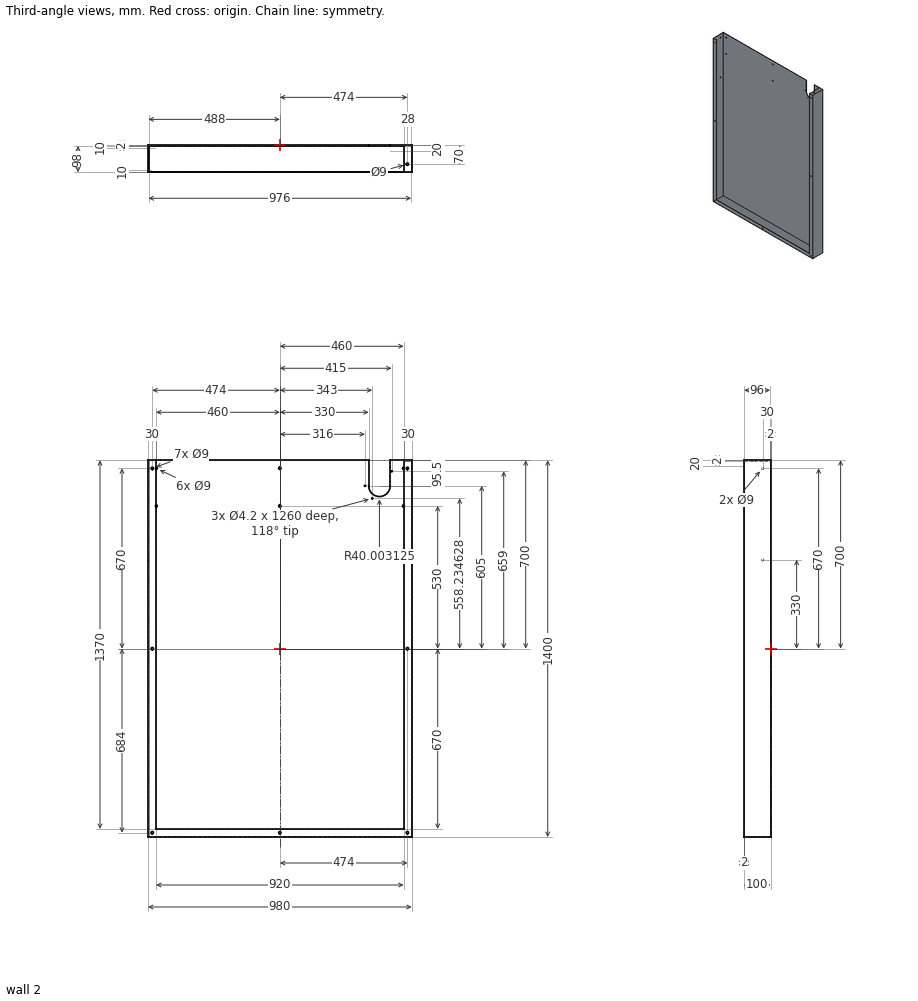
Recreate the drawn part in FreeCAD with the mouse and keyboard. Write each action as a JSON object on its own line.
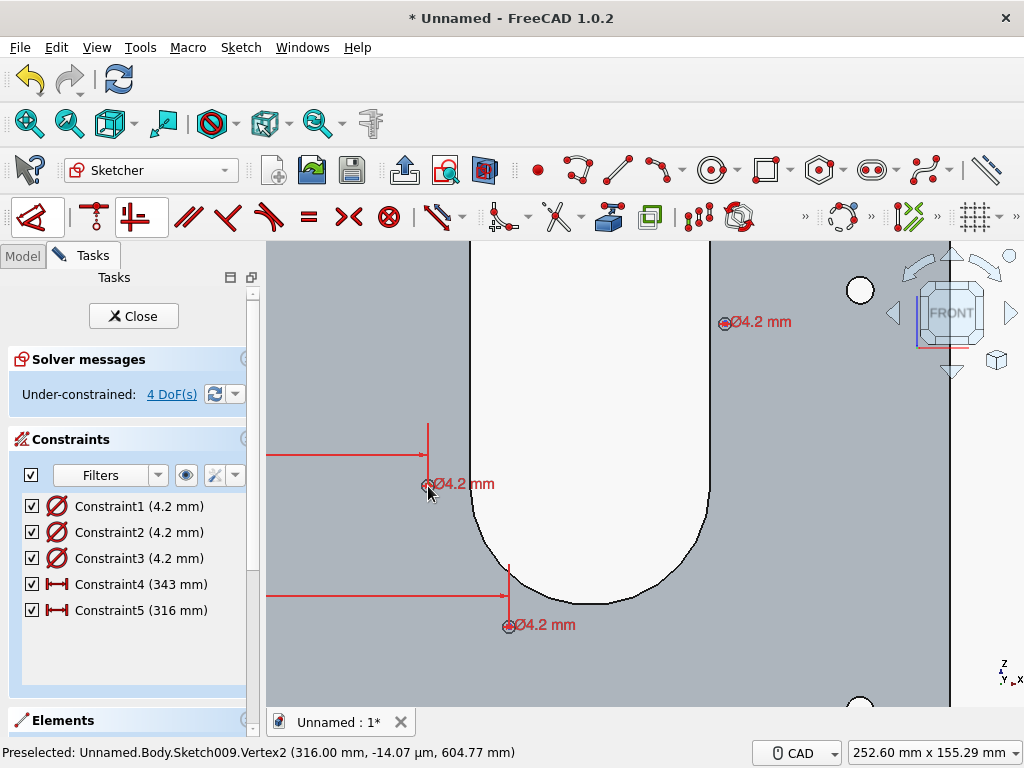
{"action": "left_click", "coordinate": [58, 218]}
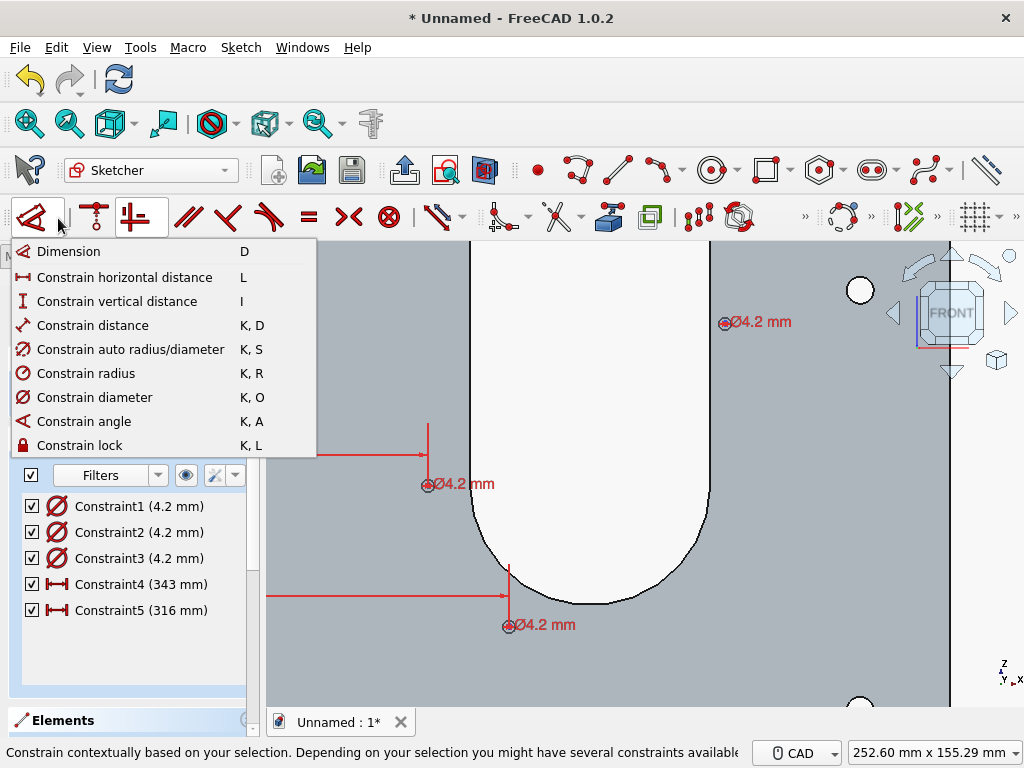
{"action": "left_click", "coordinate": [164, 301]}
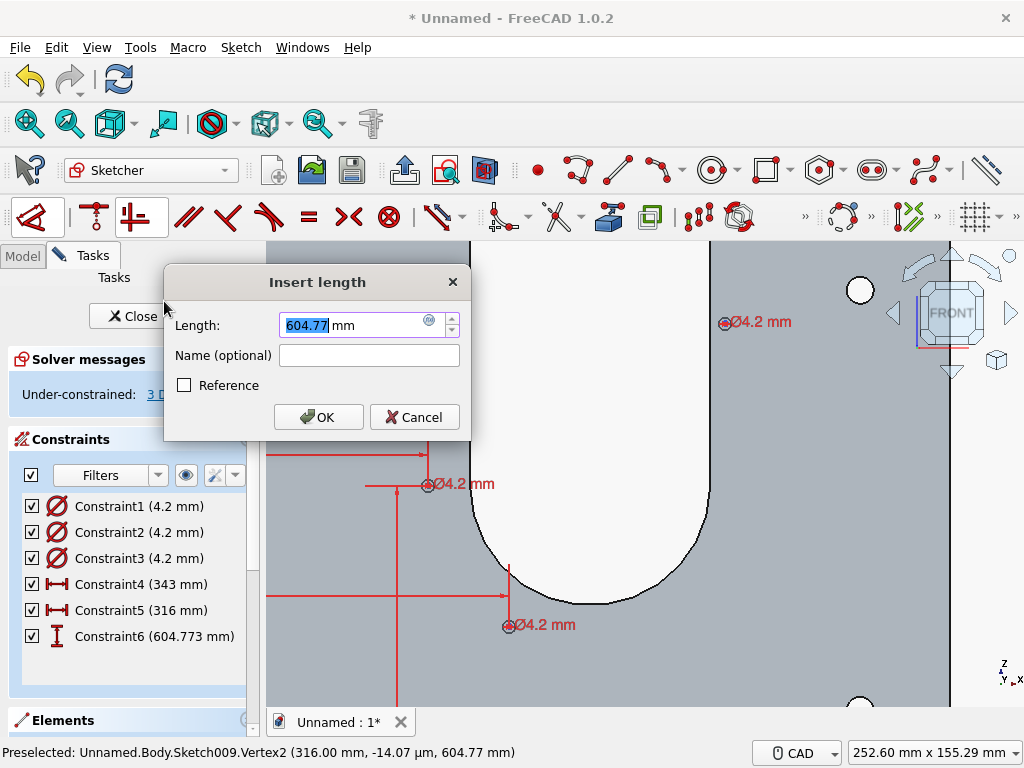
{"action": "type", "text": "605"}
{"action": "key", "text": "Return"}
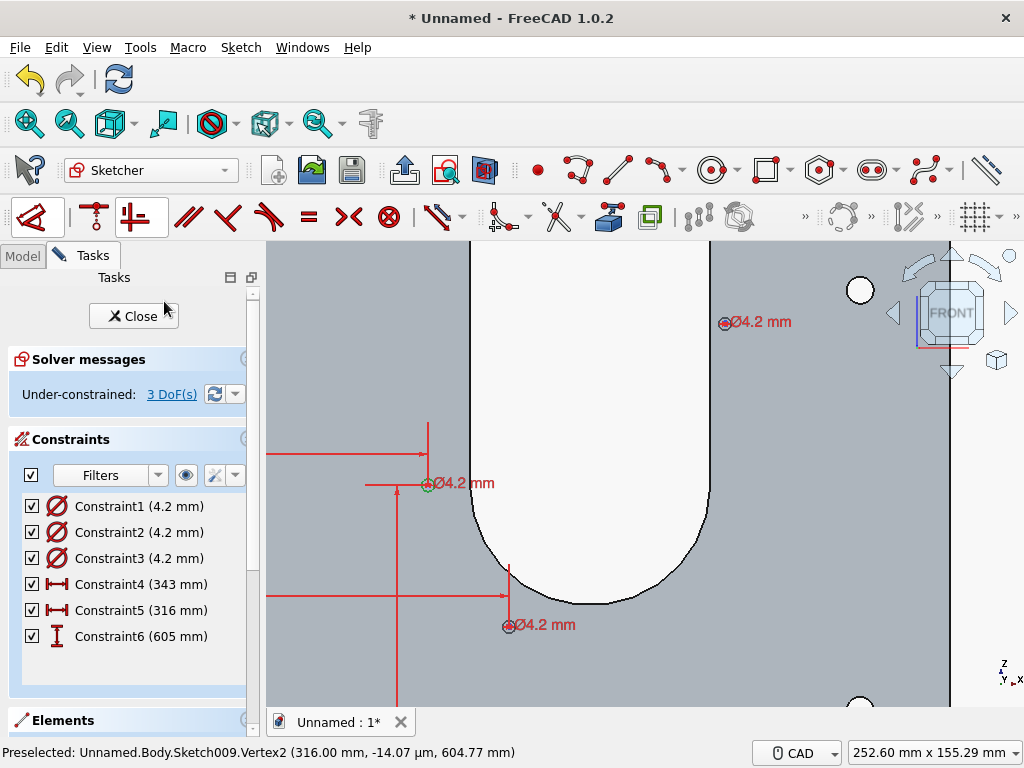
{"action": "left_click", "coordinate": [725, 324]}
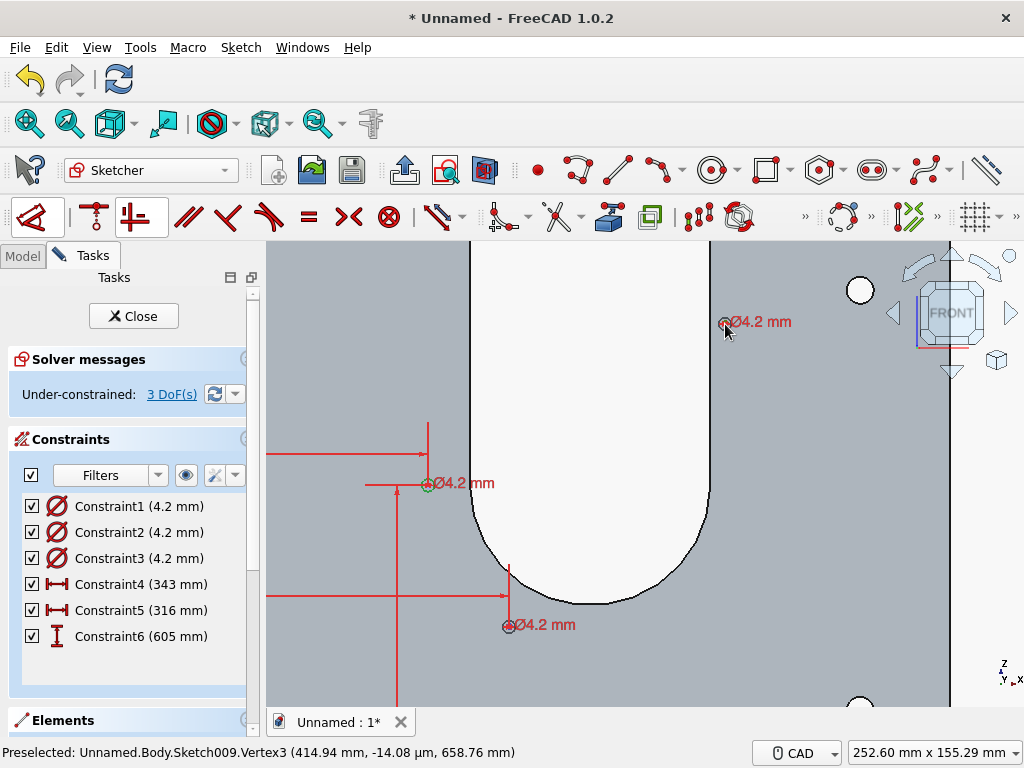
{"action": "left_click", "coordinate": [58, 218]}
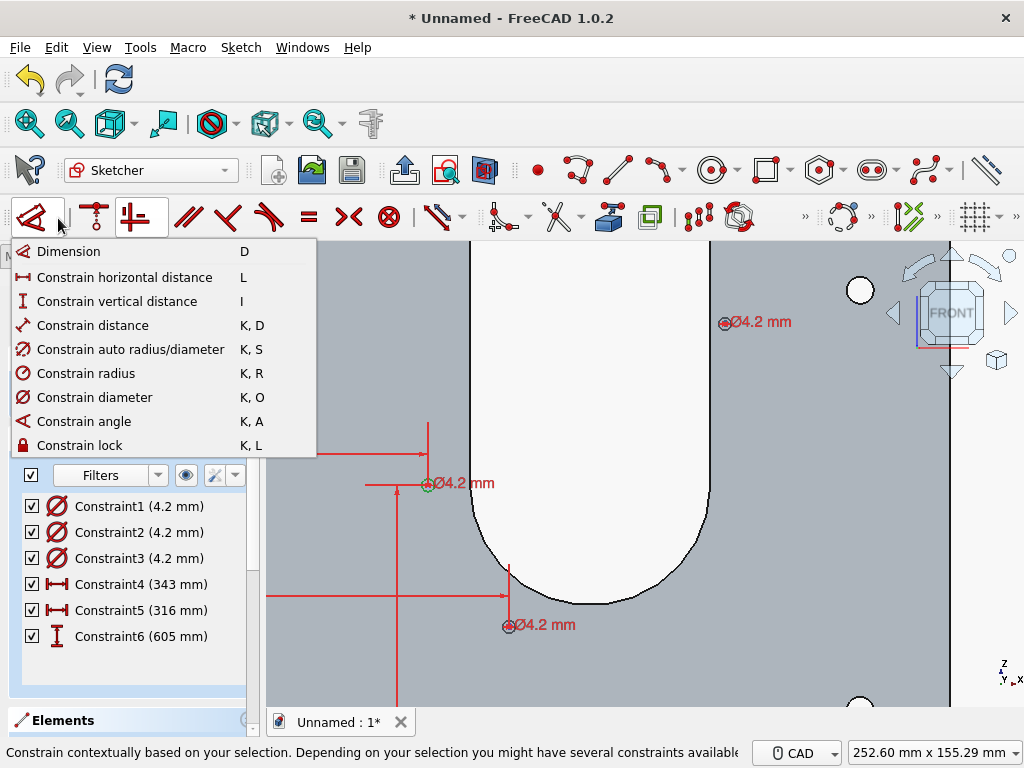
{"action": "left_click", "coordinate": [164, 277]}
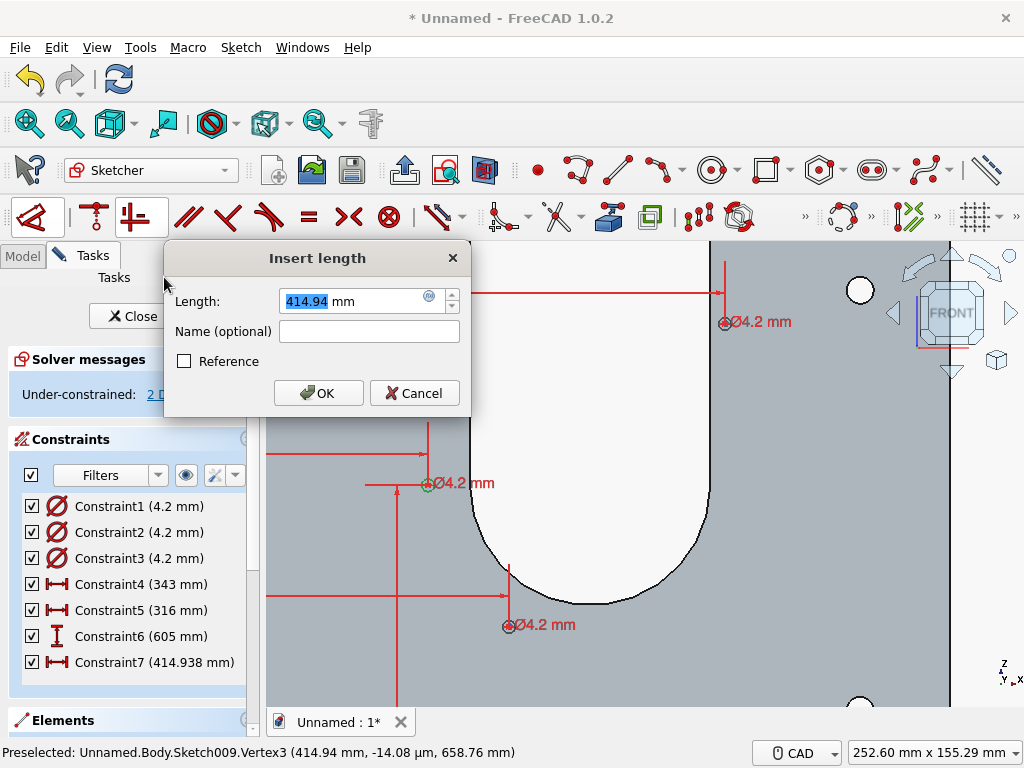
{"action": "type", "text": "415"}
{"action": "key", "text": "Return"}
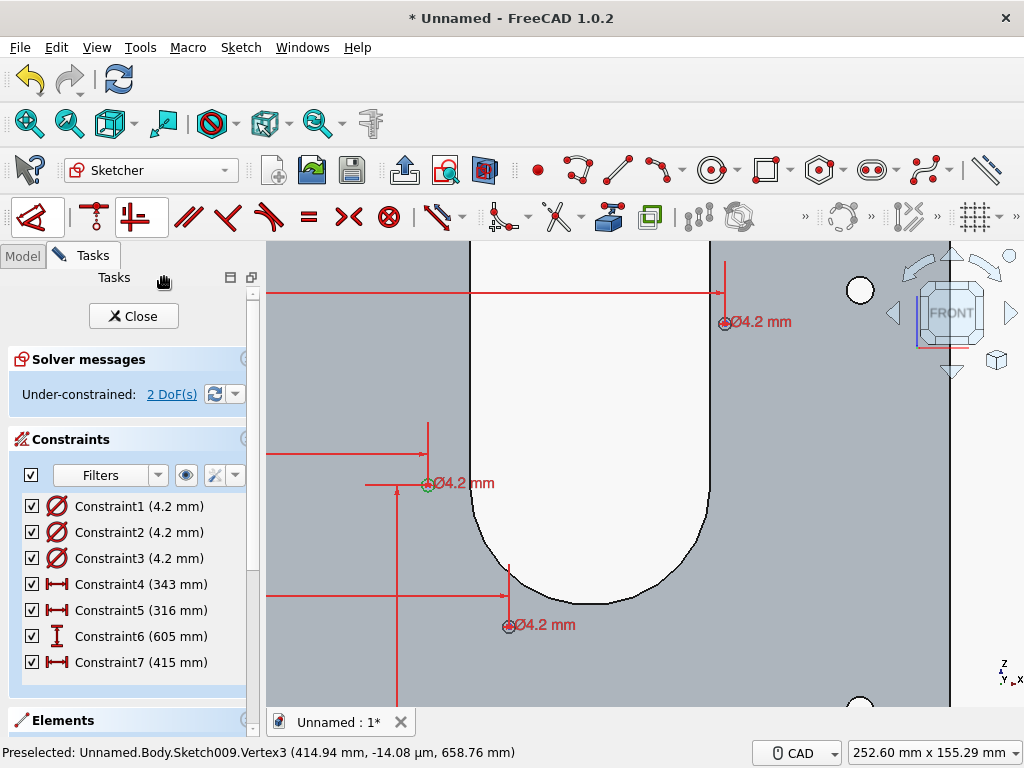
{"action": "left_click", "coordinate": [725, 324]}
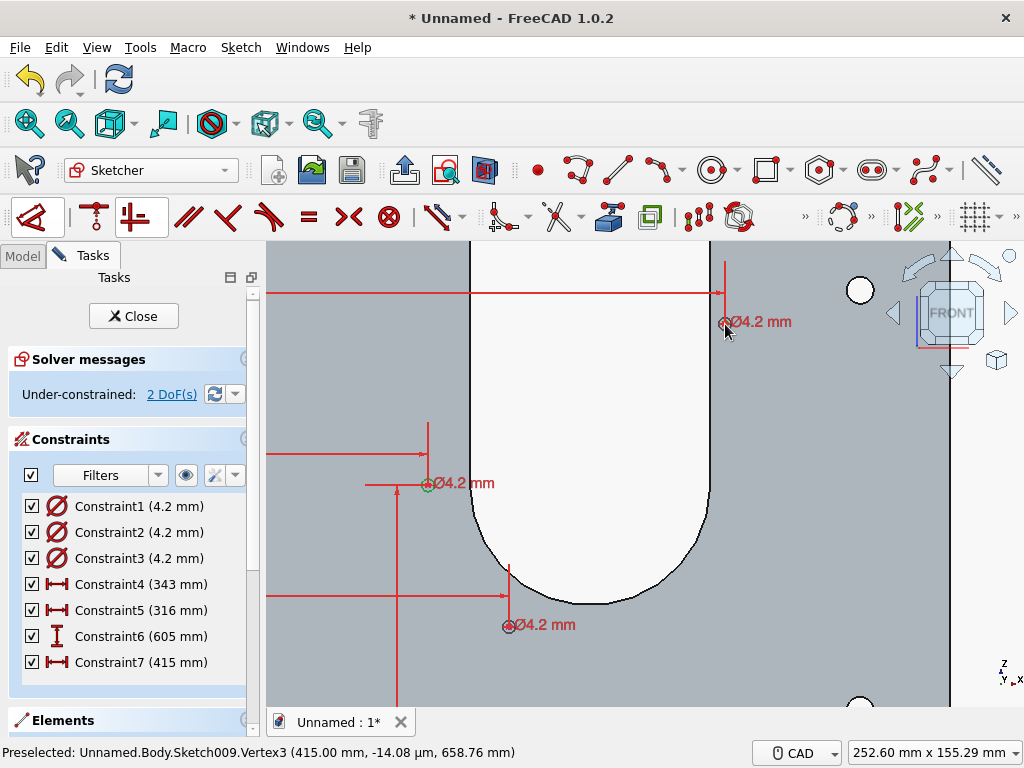
{"action": "left_click", "coordinate": [58, 218]}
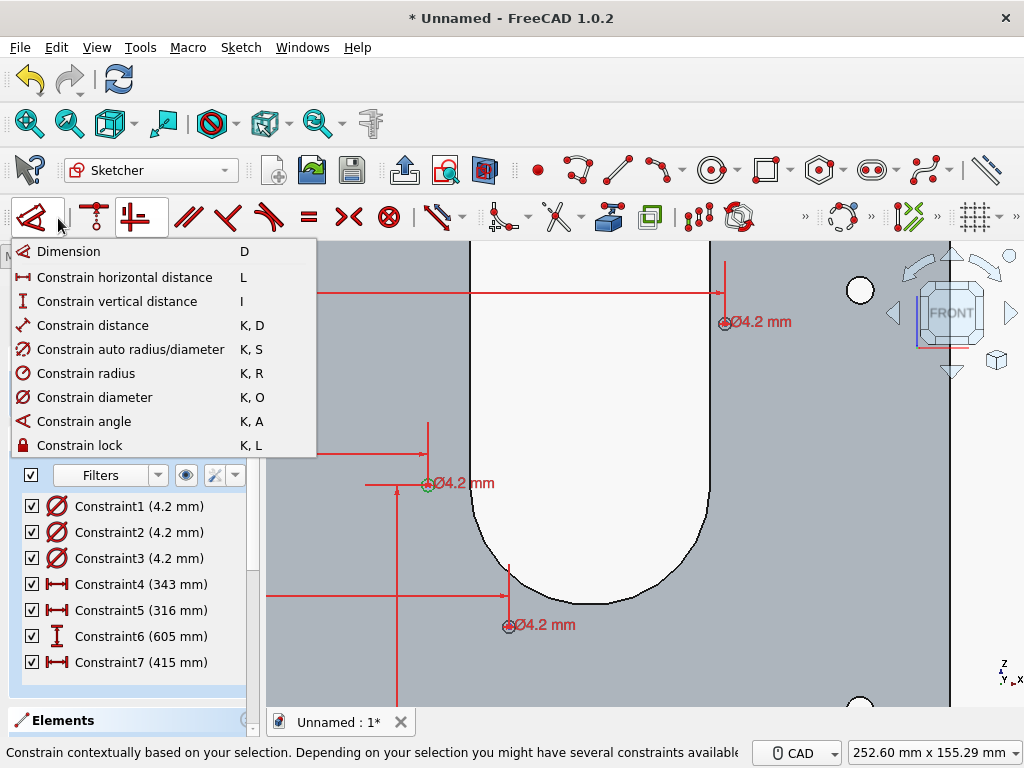
{"action": "left_click", "coordinate": [164, 301]}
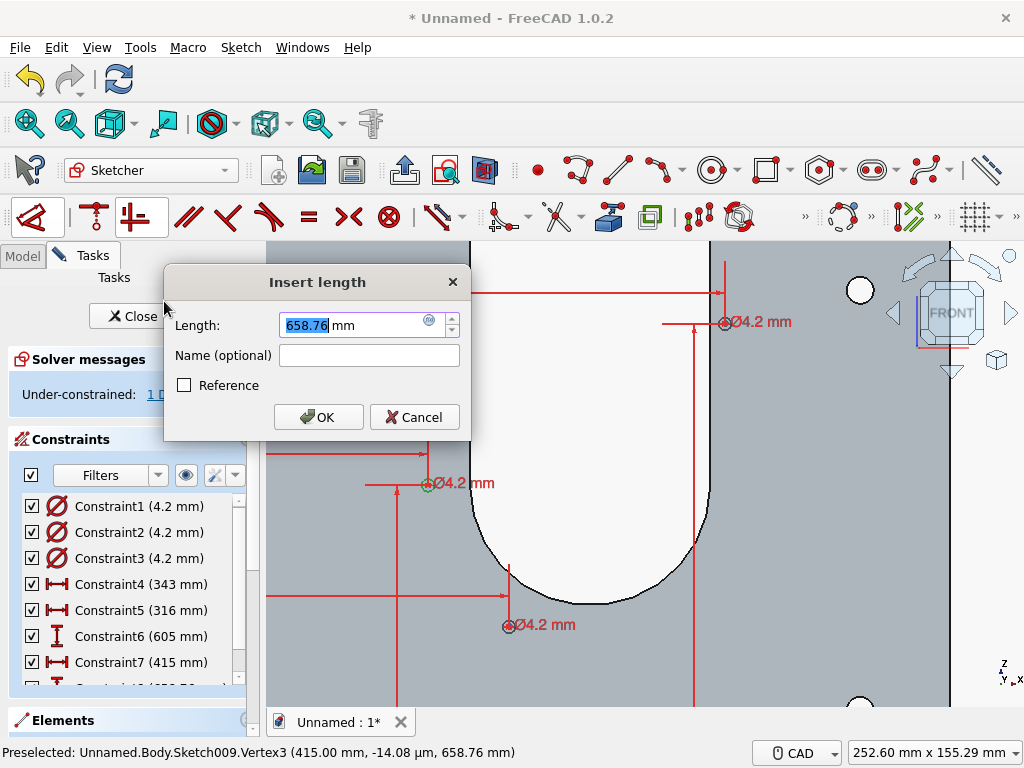
{"action": "type", "text": "659"}
{"action": "key", "text": "Return"}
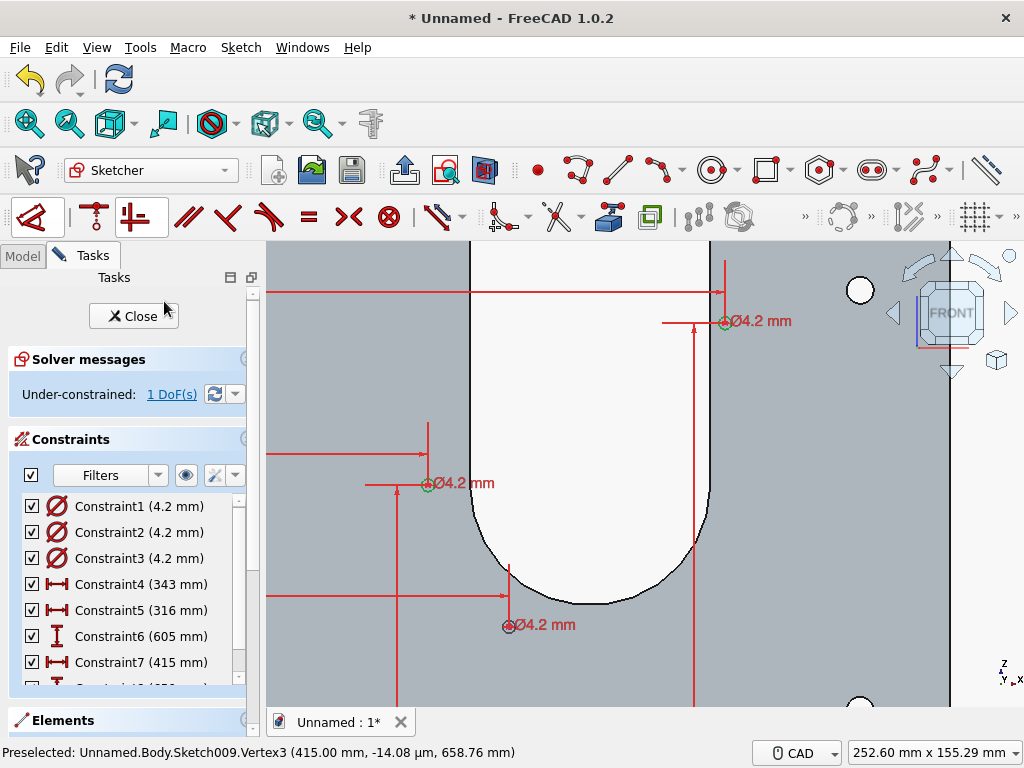
{"action": "left_click", "coordinate": [509, 627]}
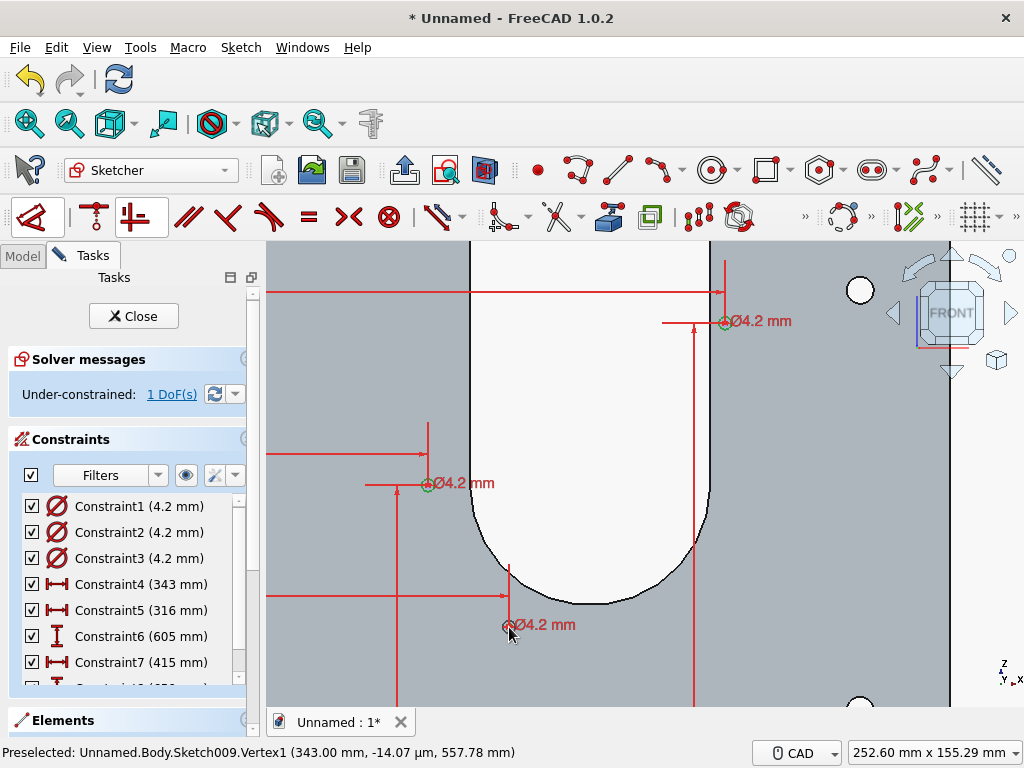
{"action": "left_click", "coordinate": [58, 218]}